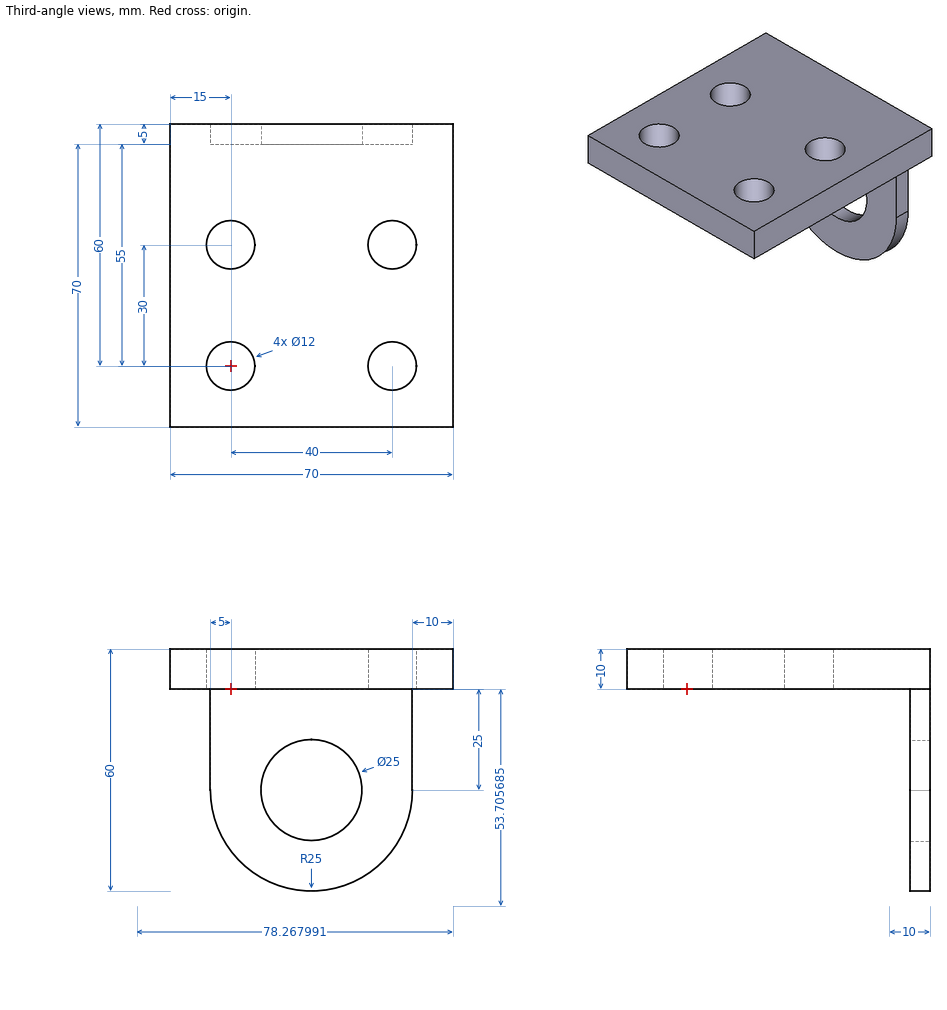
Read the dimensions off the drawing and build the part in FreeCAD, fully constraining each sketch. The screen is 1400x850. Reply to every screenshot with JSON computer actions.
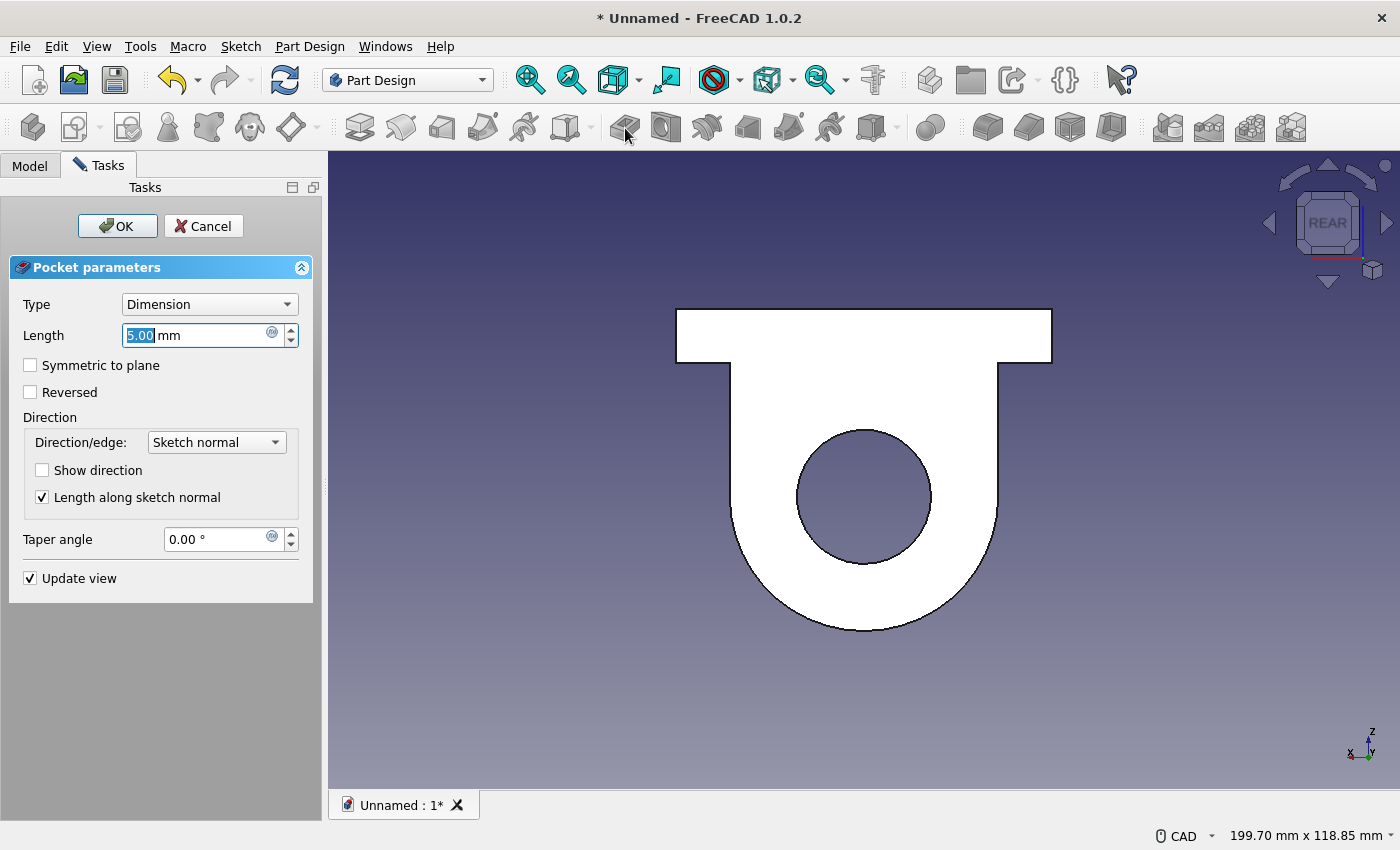
{"action": "type", "text": "10"}
{"action": "key", "text": "Tab"}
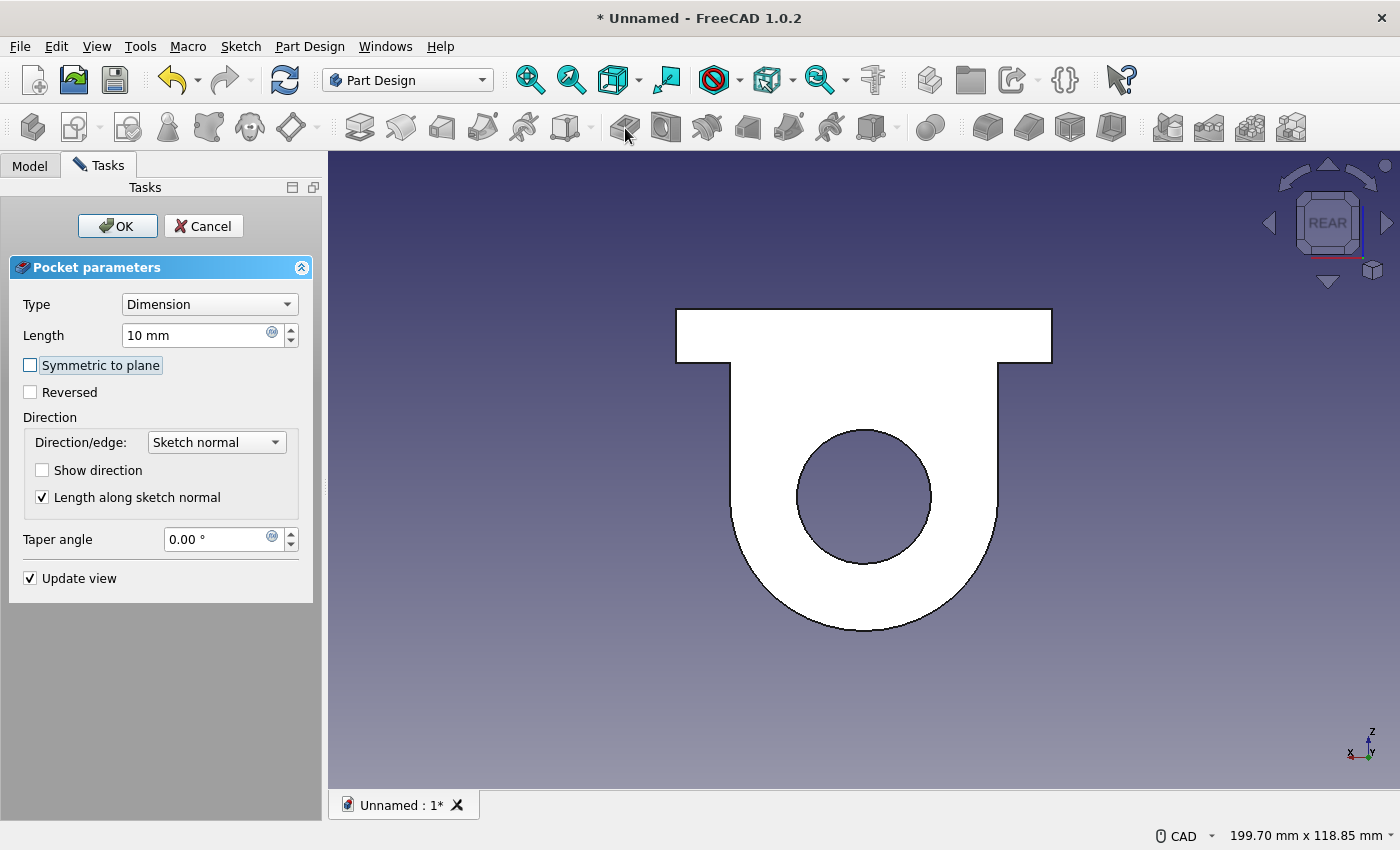
{"action": "left_click", "coordinate": [118, 226]}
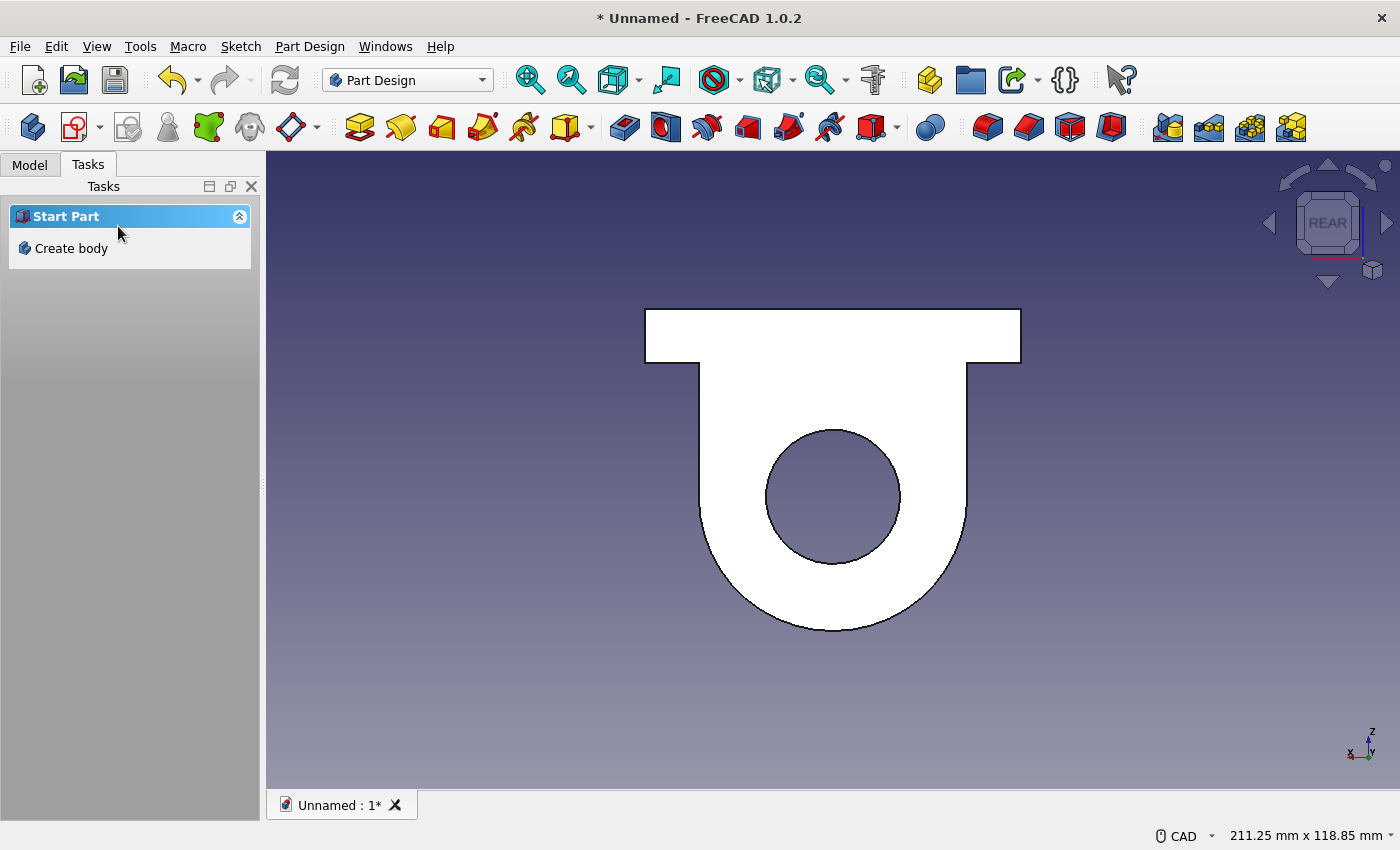
{"action": "key", "text": "0"}